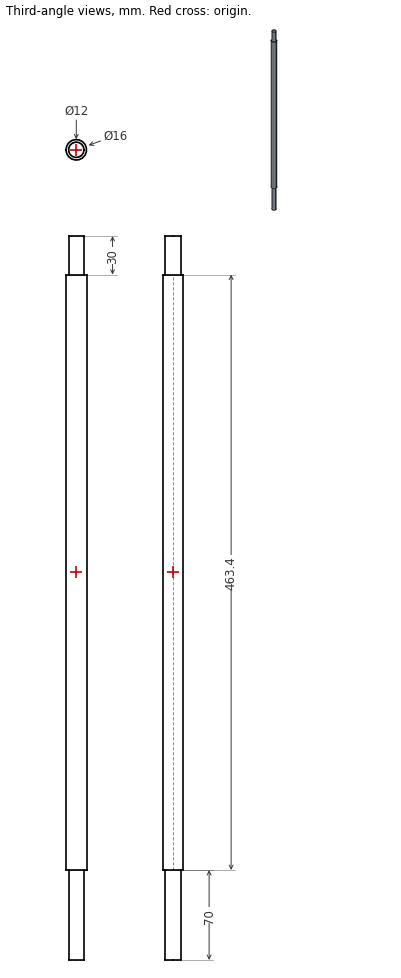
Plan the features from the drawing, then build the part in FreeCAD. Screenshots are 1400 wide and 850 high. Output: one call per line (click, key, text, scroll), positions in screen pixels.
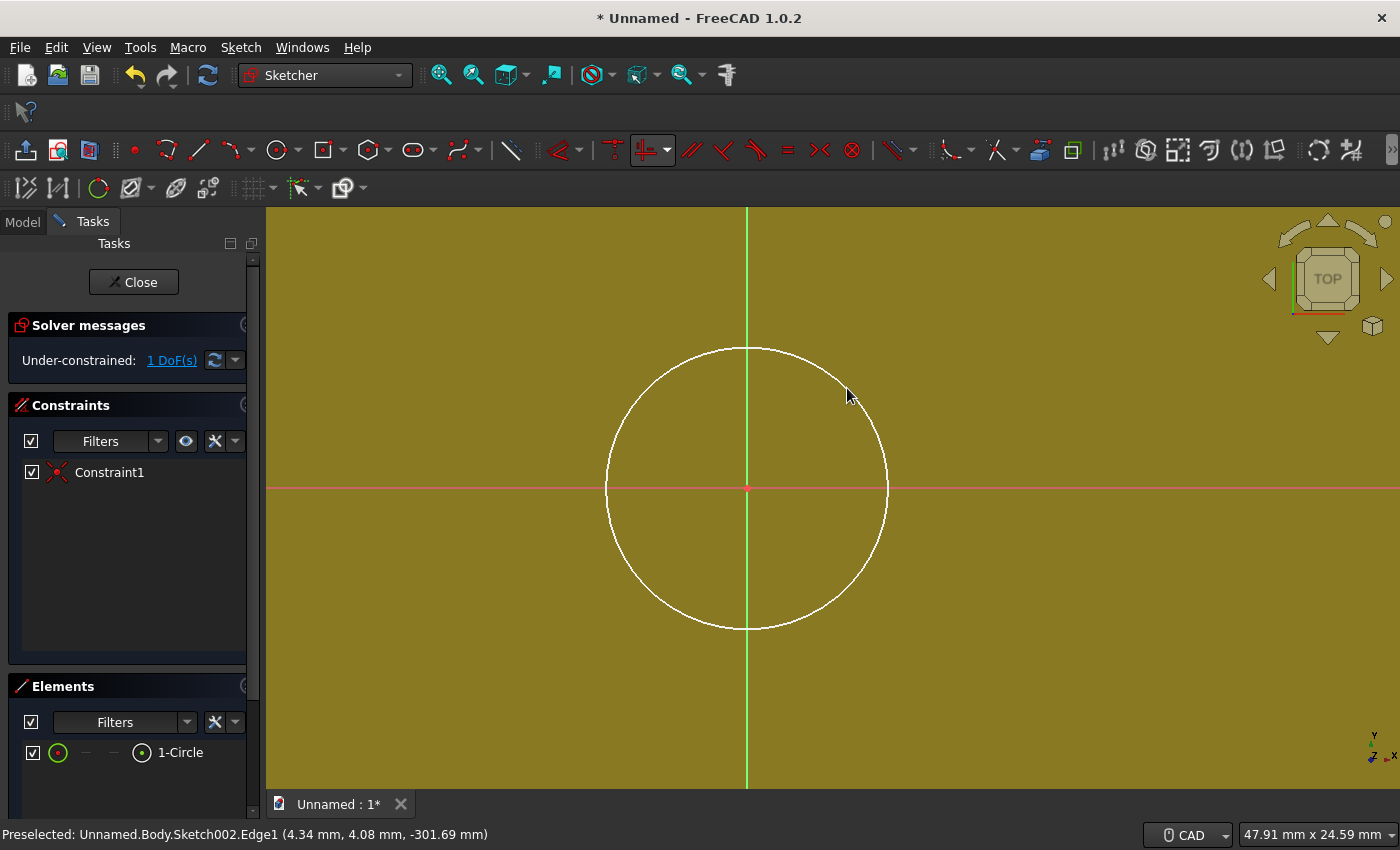
key(d)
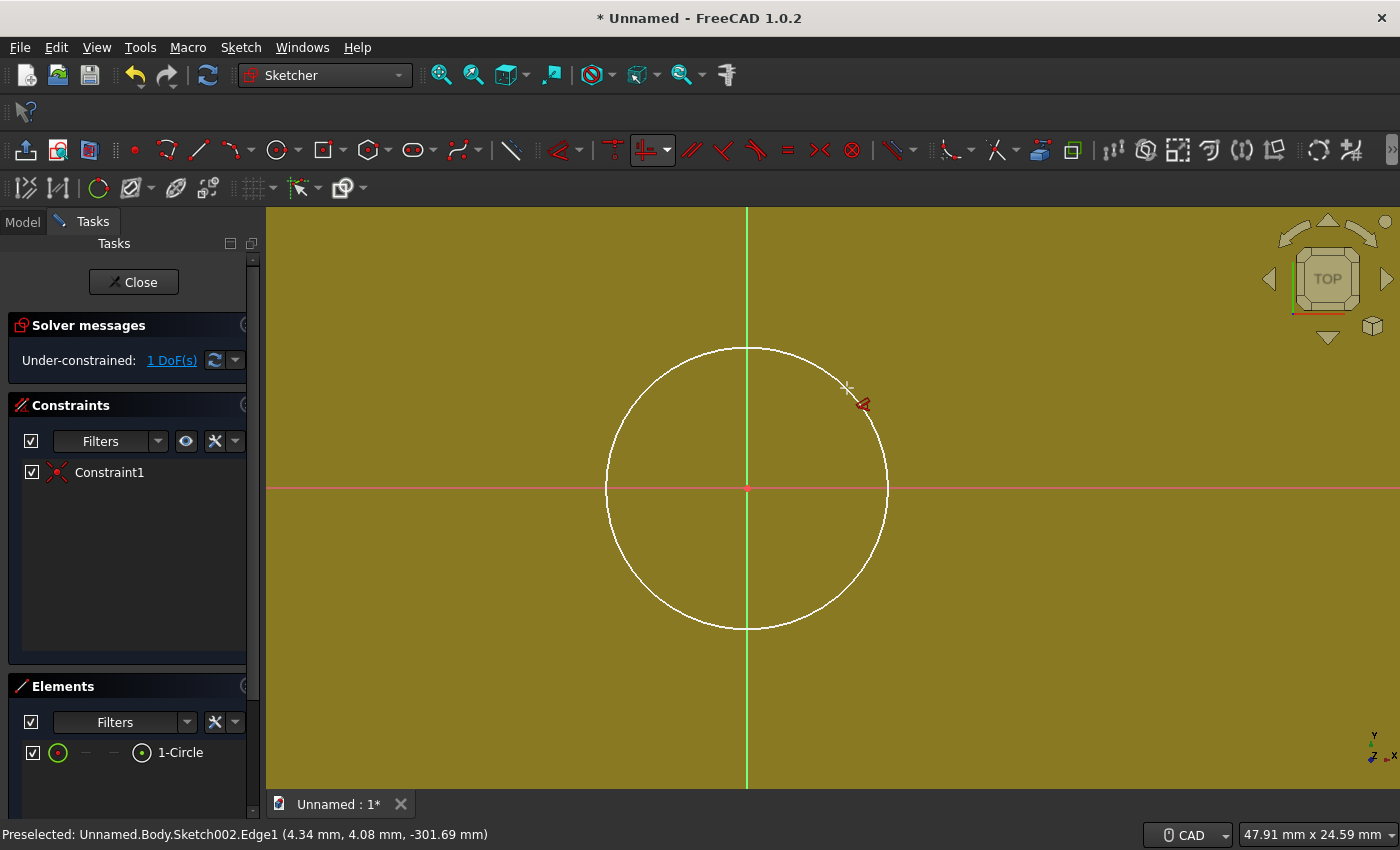
click(846, 388)
click(868, 365)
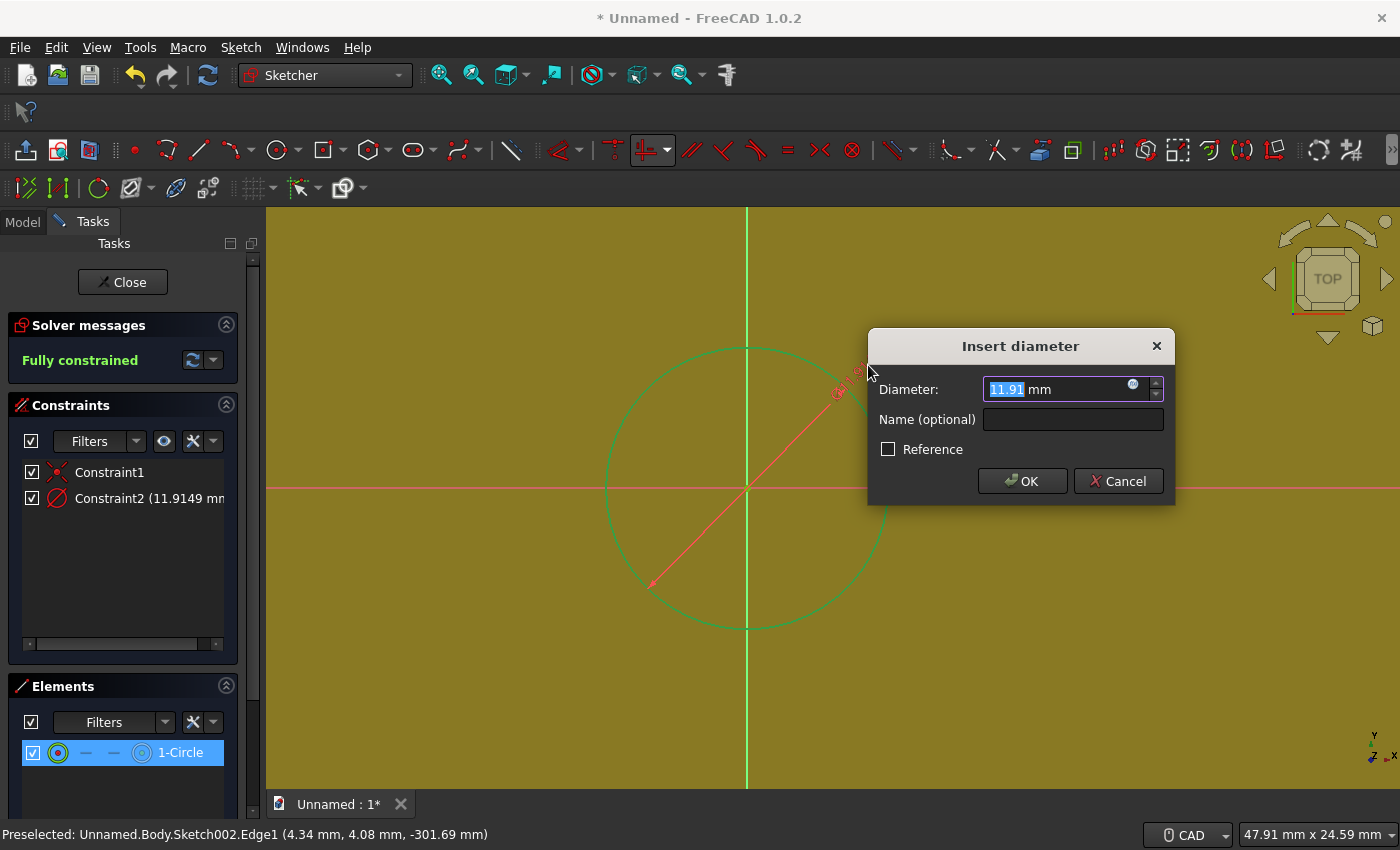
text(12)
key(Return)
key(Escape)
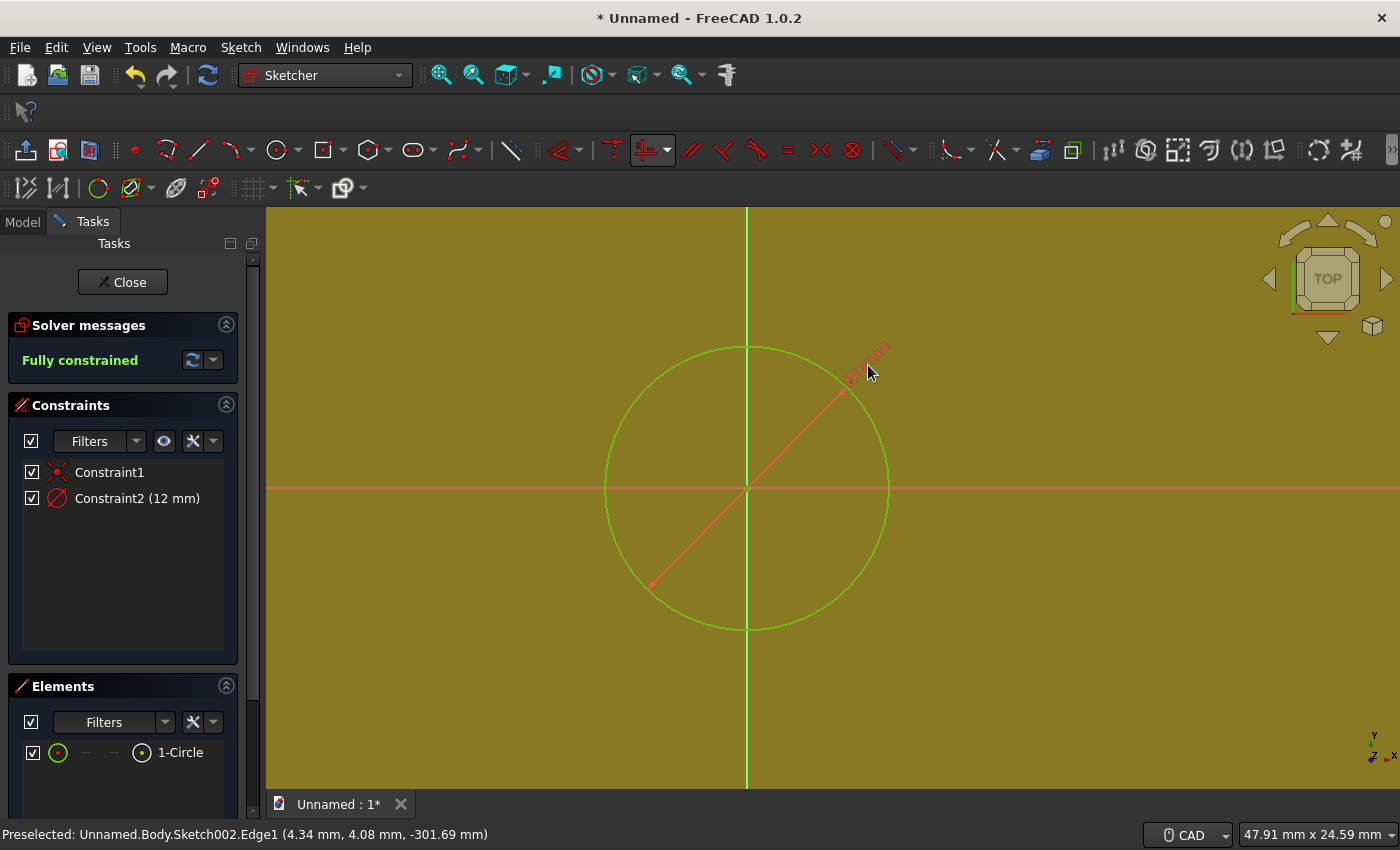
click(123, 282)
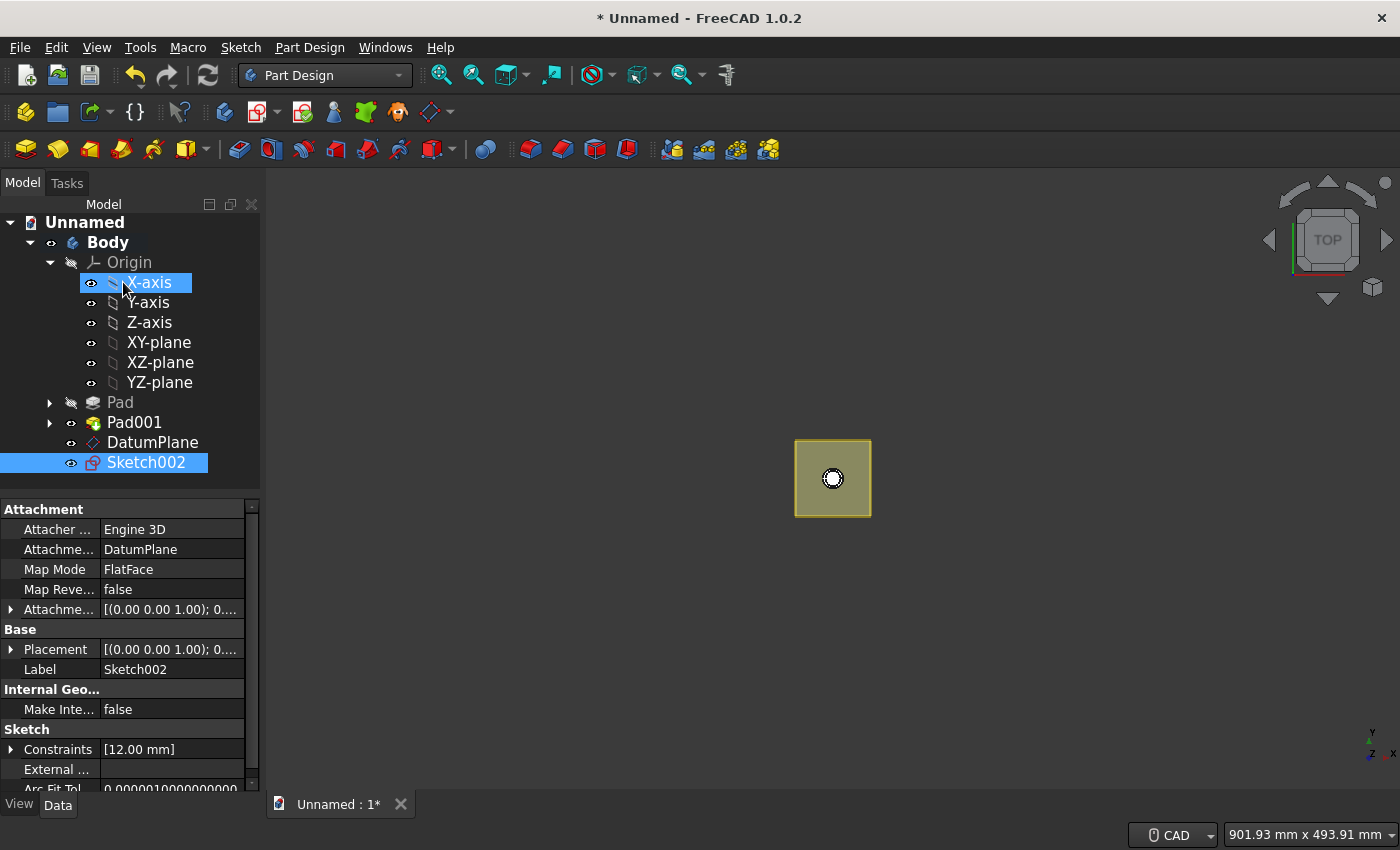
click(26, 150)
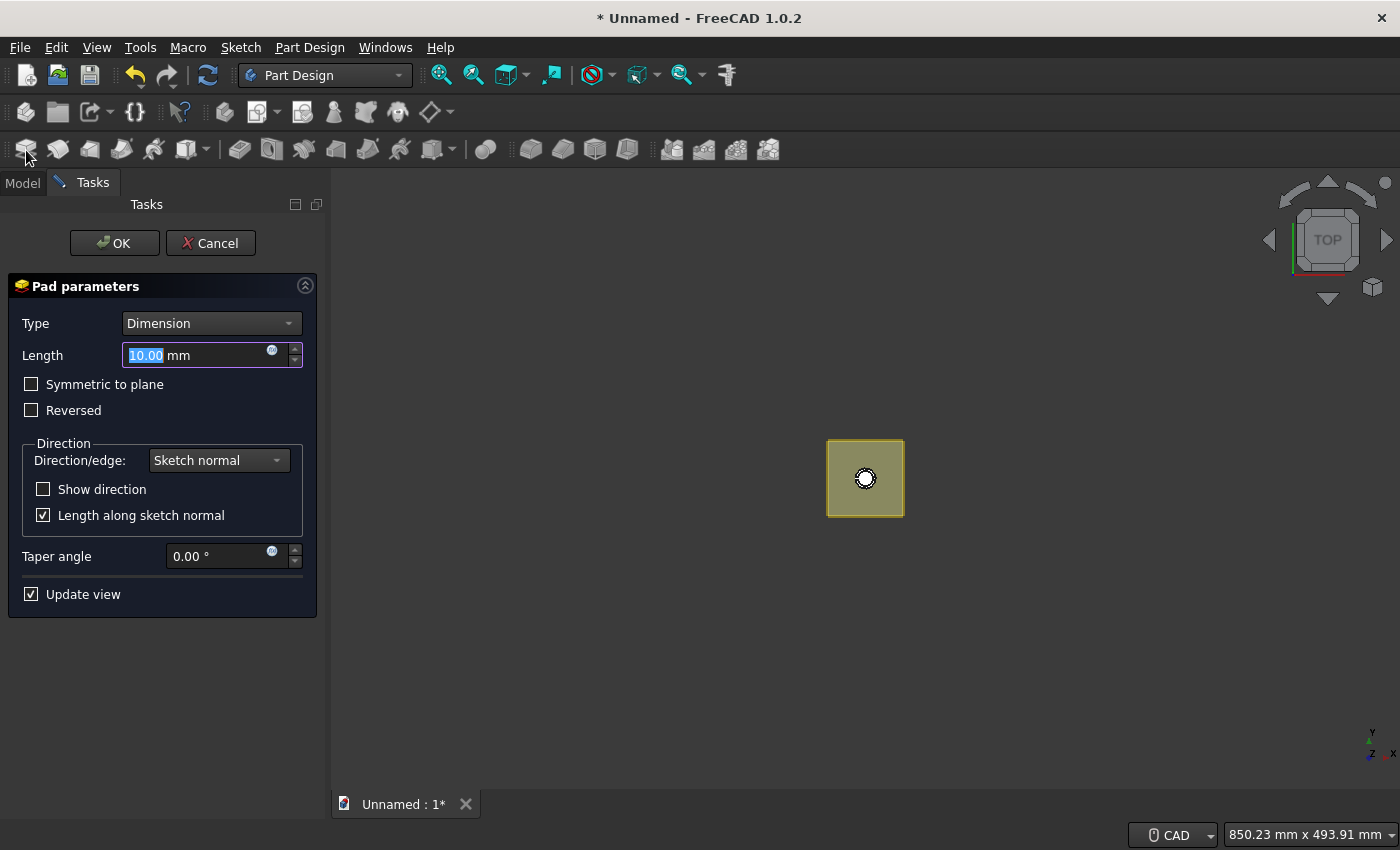
text(70)
key(Tab)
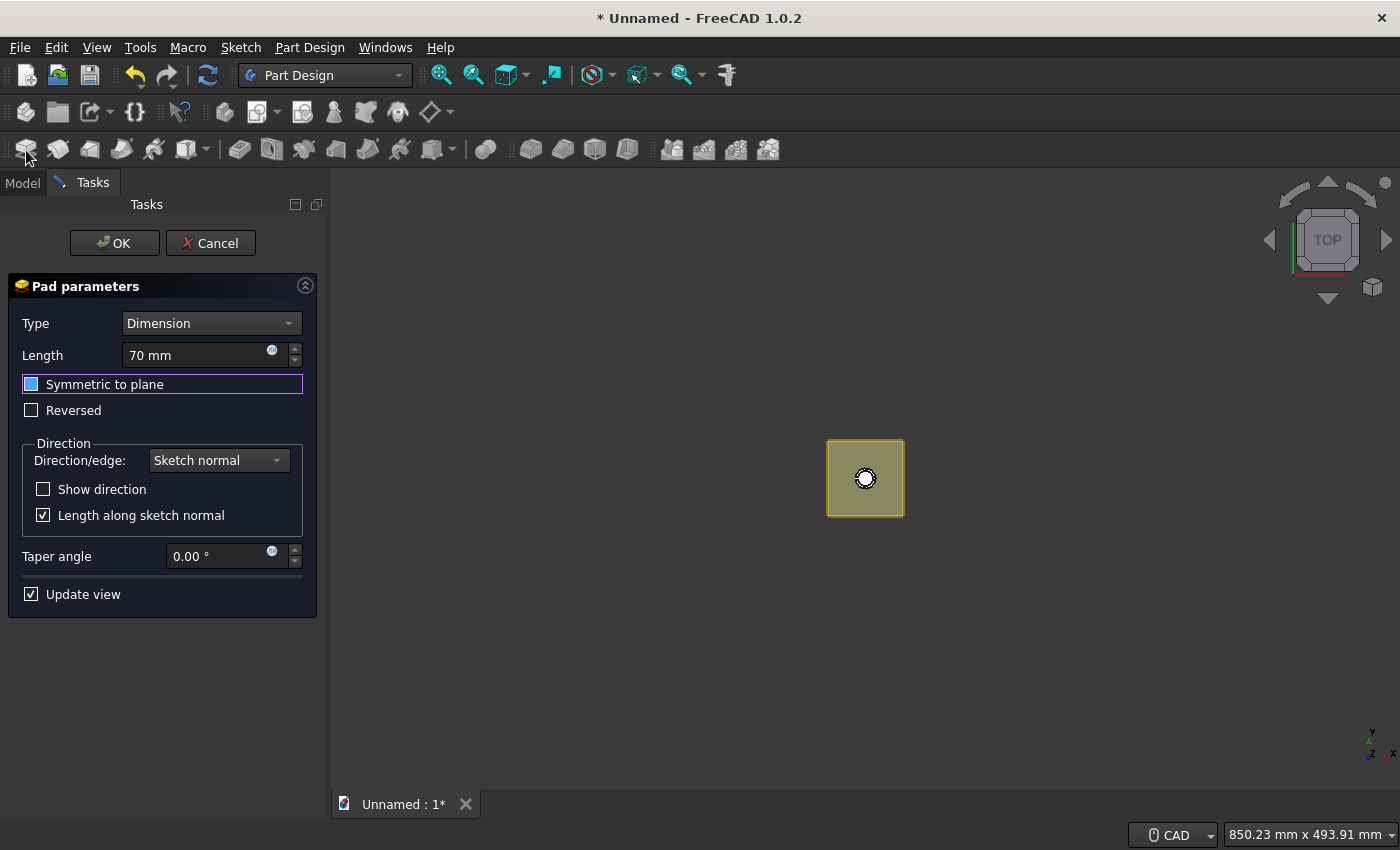
click(115, 243)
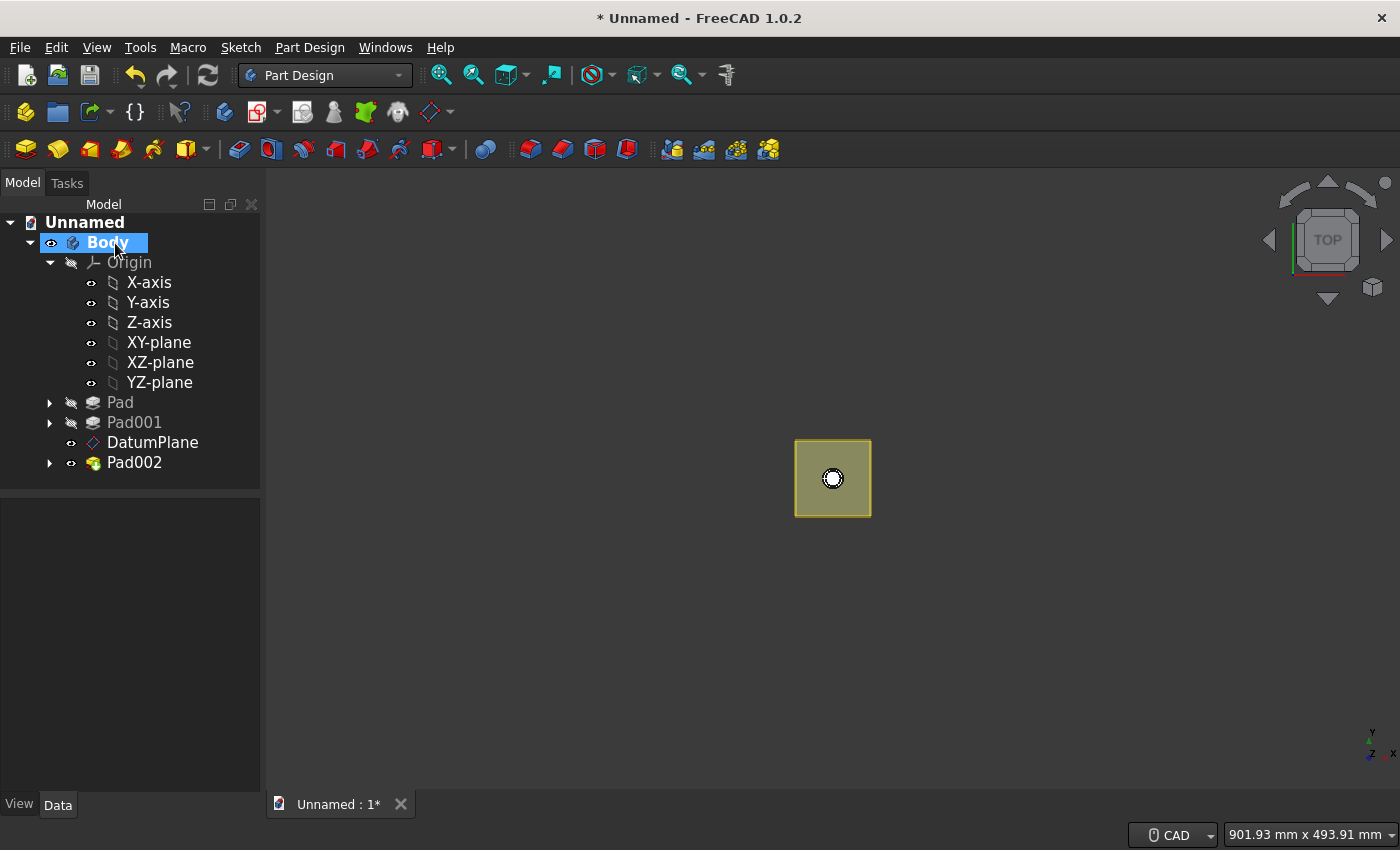
click(116, 443)
key(space)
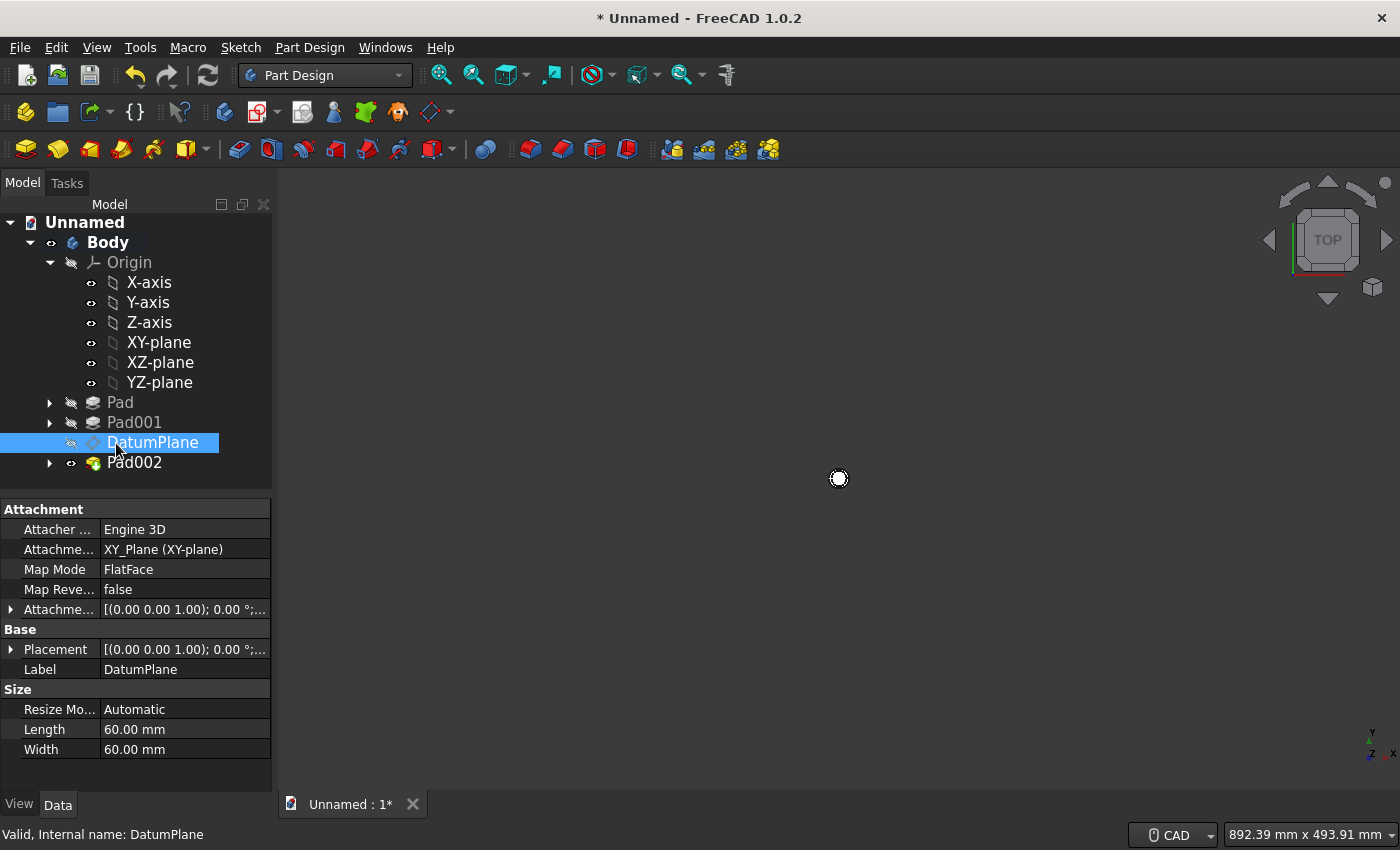
key(0)